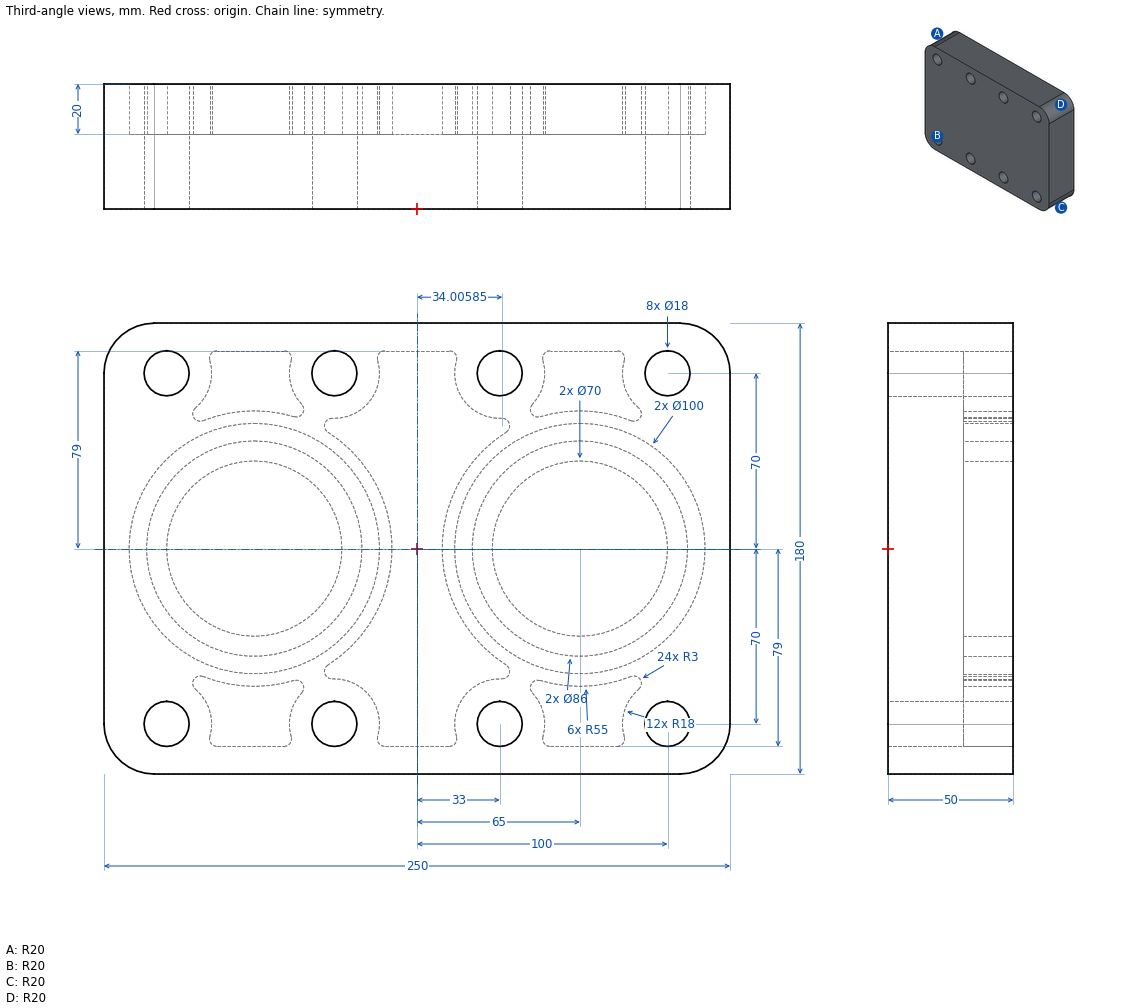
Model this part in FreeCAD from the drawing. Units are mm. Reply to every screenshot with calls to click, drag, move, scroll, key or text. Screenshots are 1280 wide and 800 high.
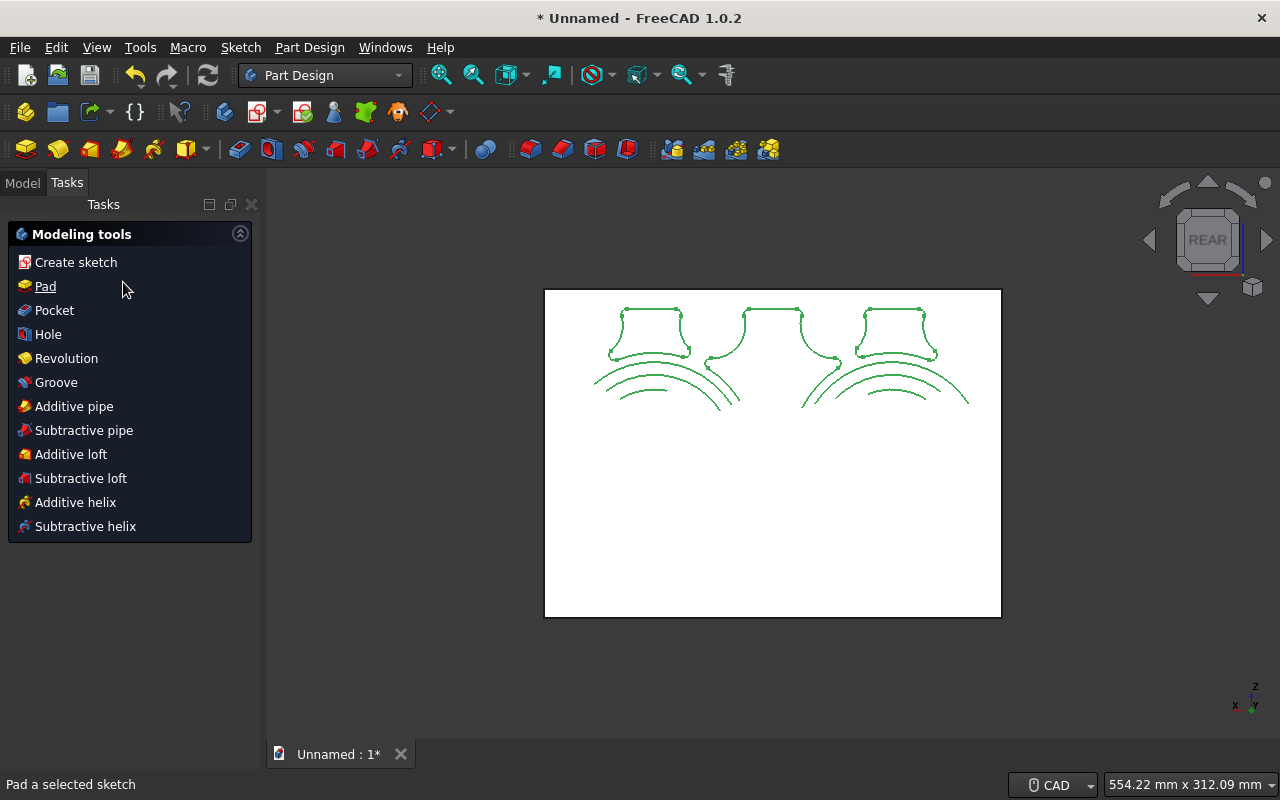
click(240, 150)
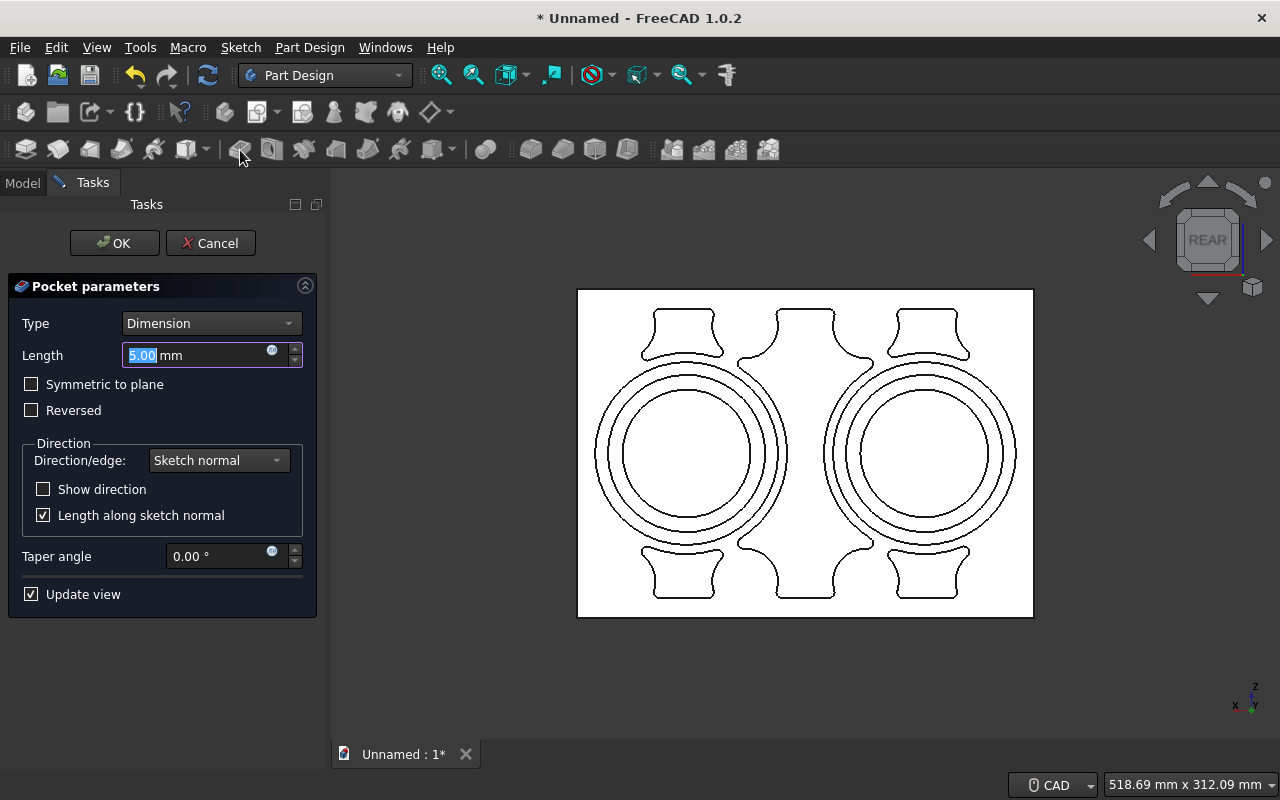
text(20)
key(Tab)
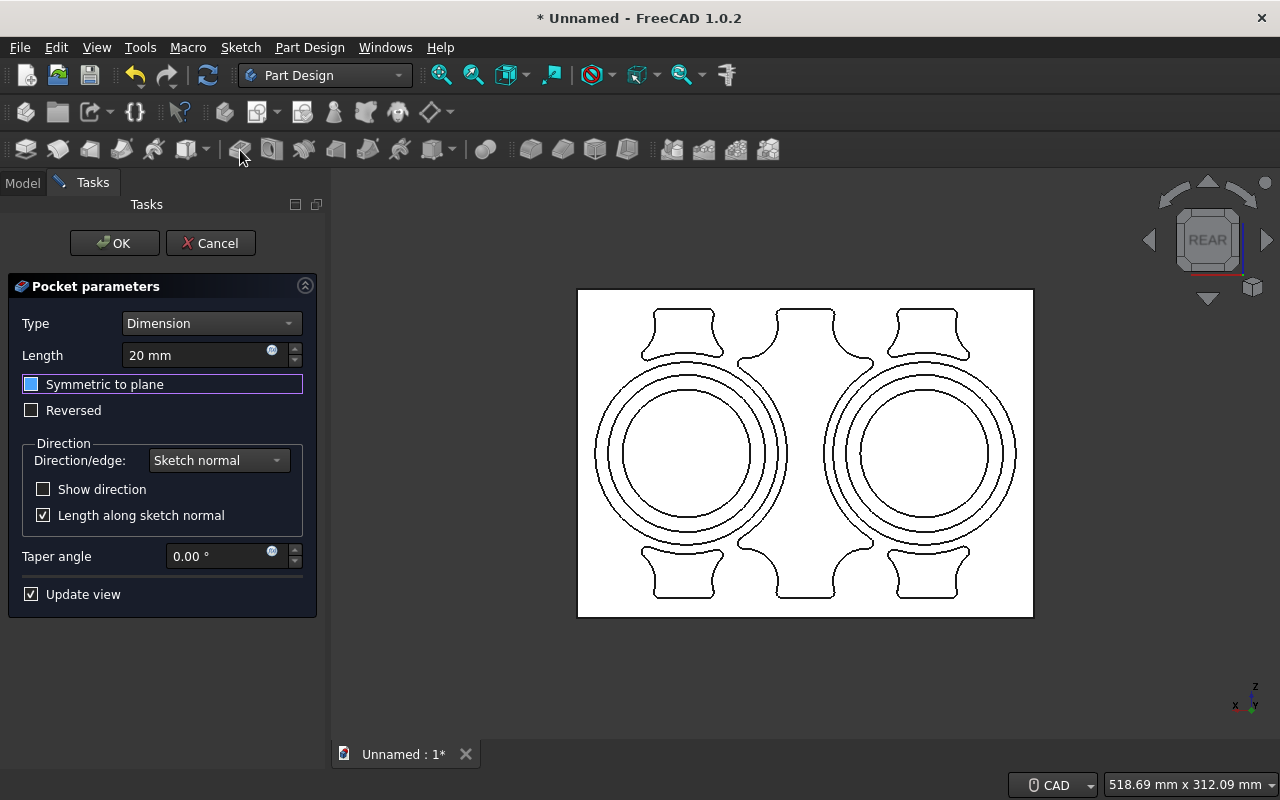
click(115, 243)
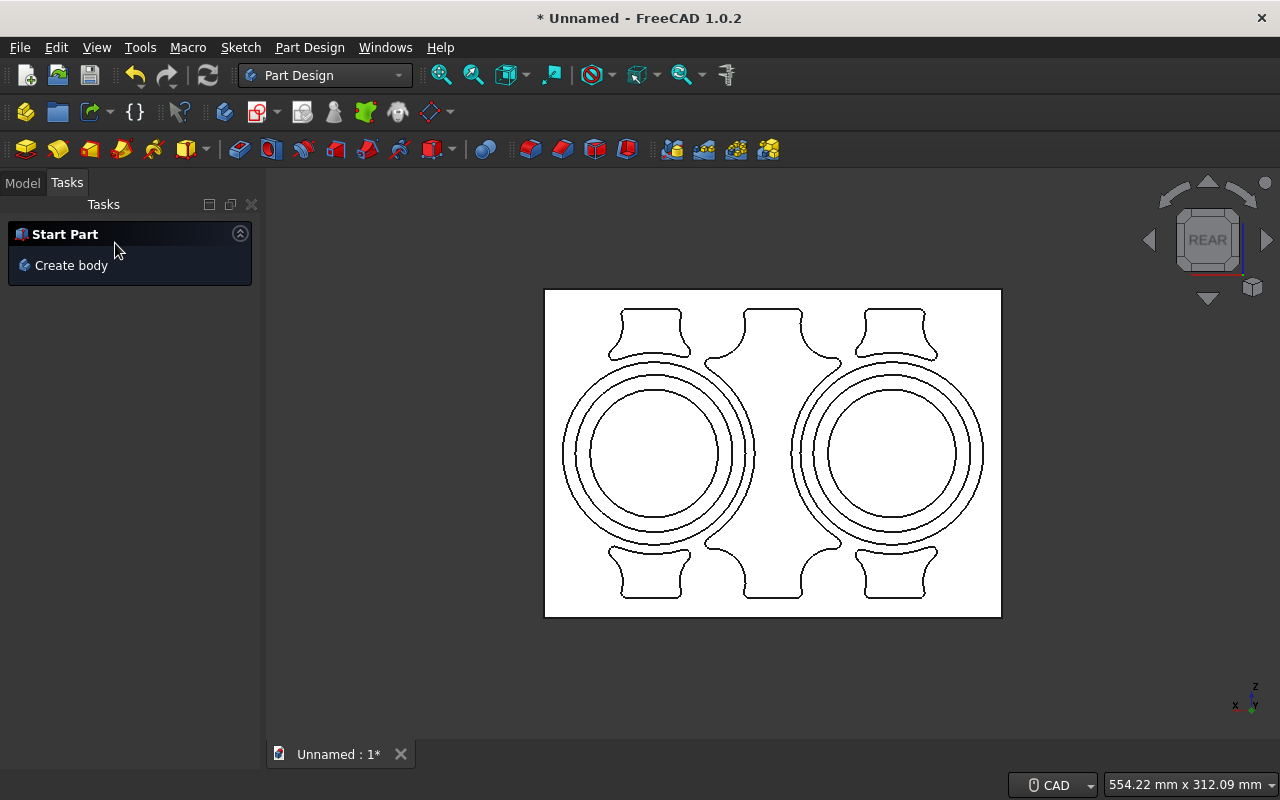
click(577, 547)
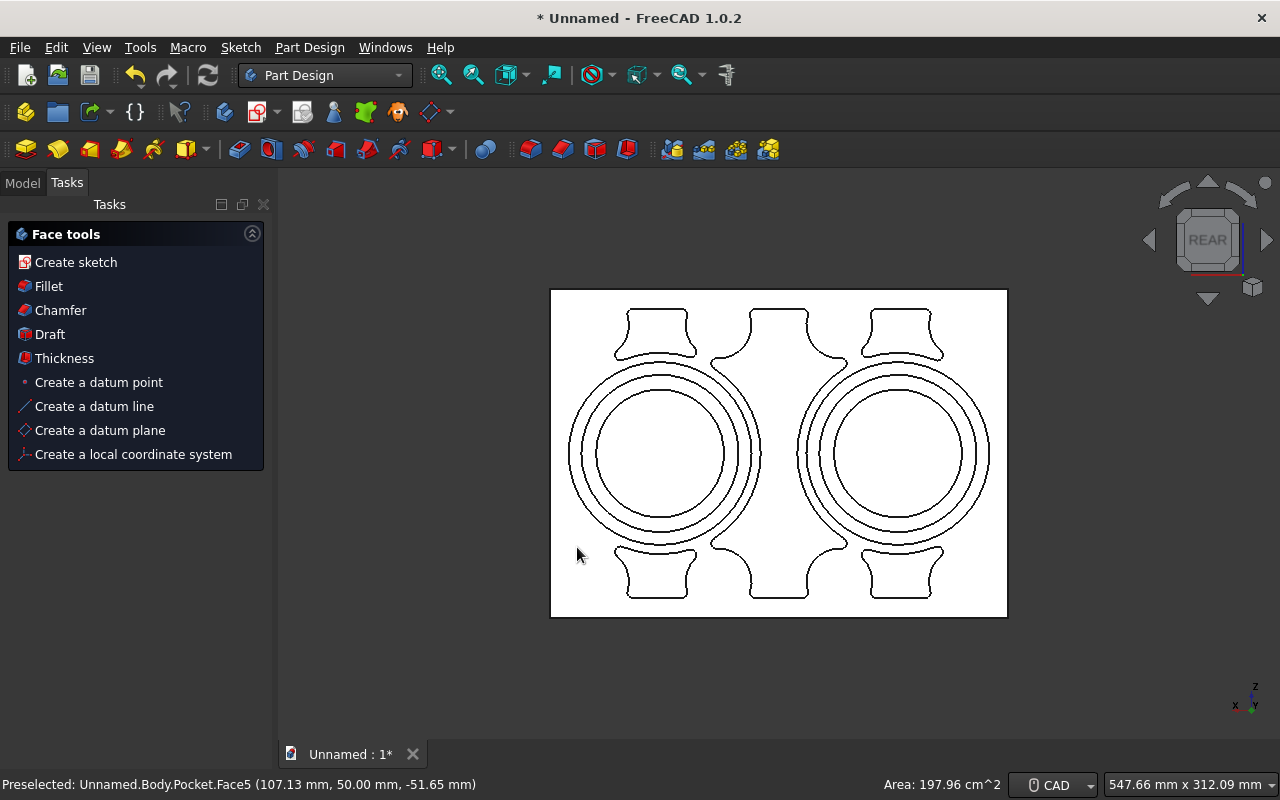
click(258, 112)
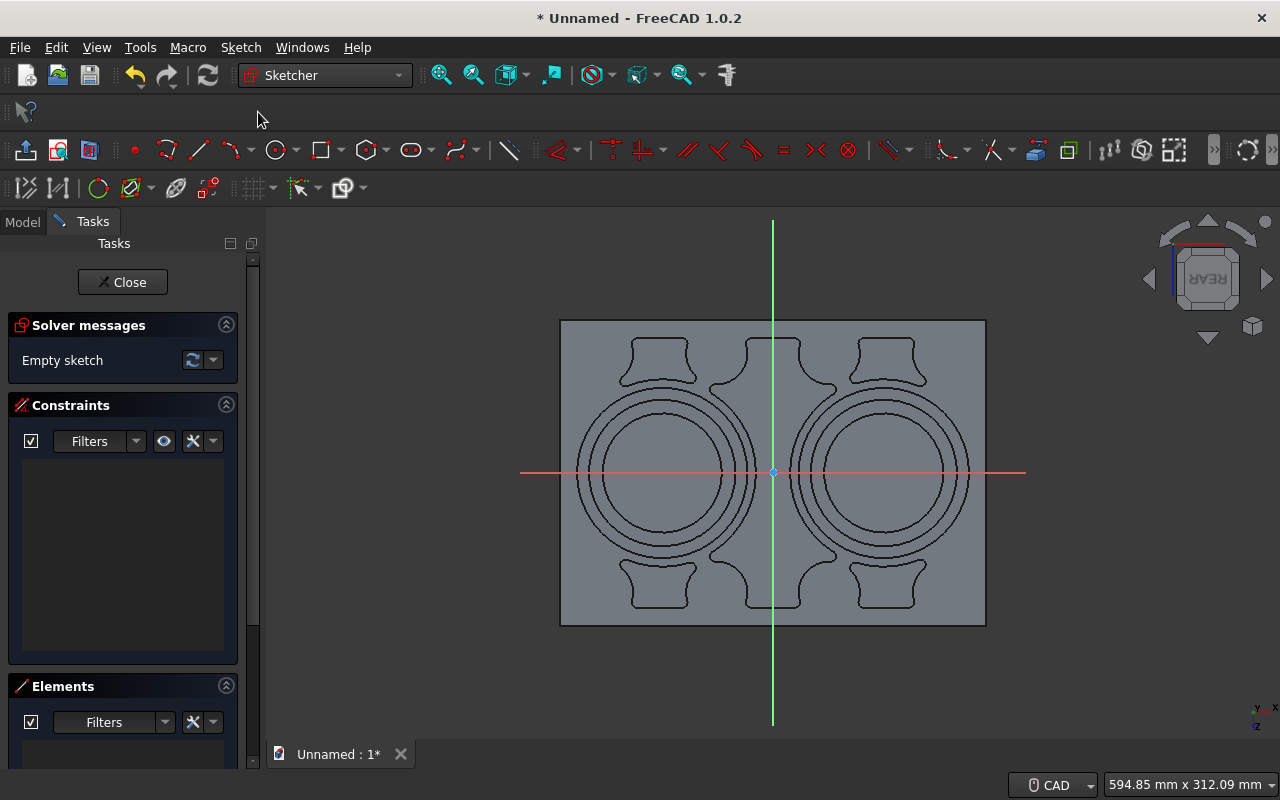
click(276, 150)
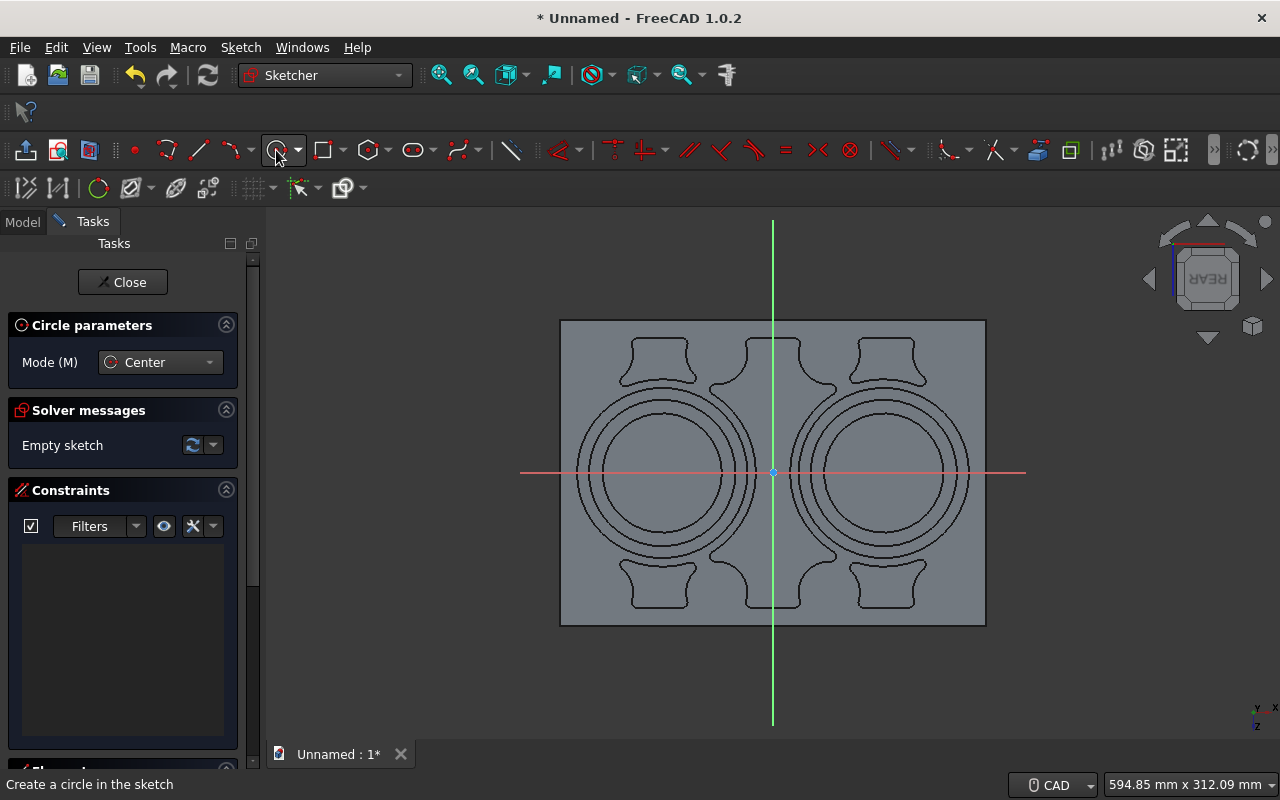
scroll(943, 592, up, 2)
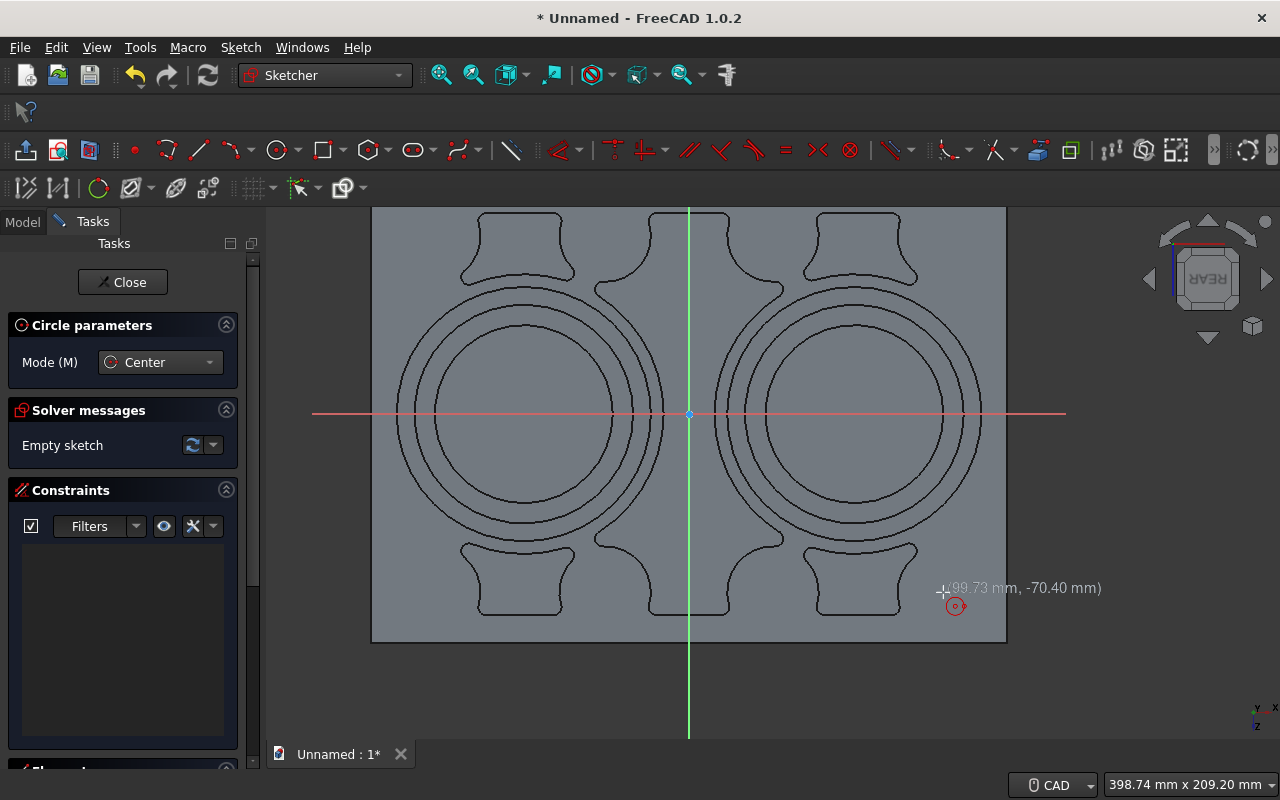
click(943, 592)
move(960, 576)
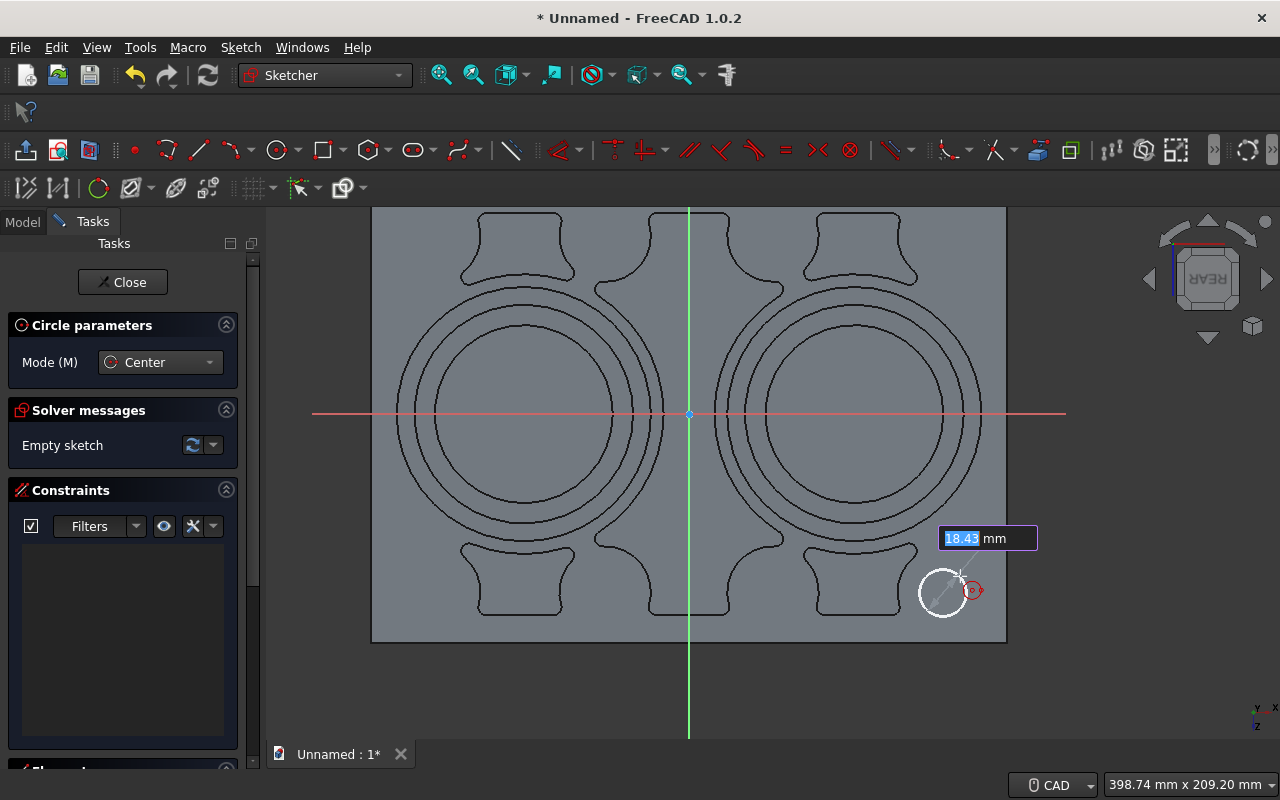
text(18)
key(Return)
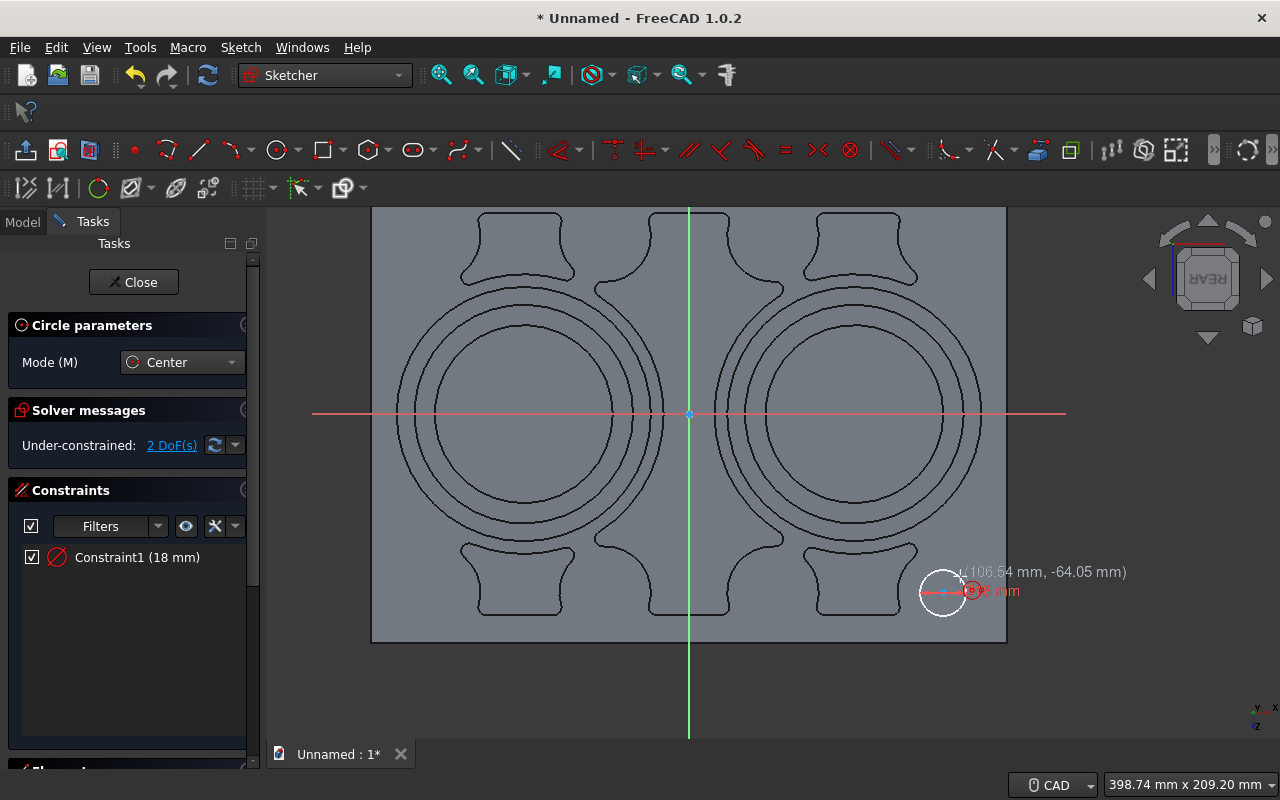
click(773, 592)
move(789, 576)